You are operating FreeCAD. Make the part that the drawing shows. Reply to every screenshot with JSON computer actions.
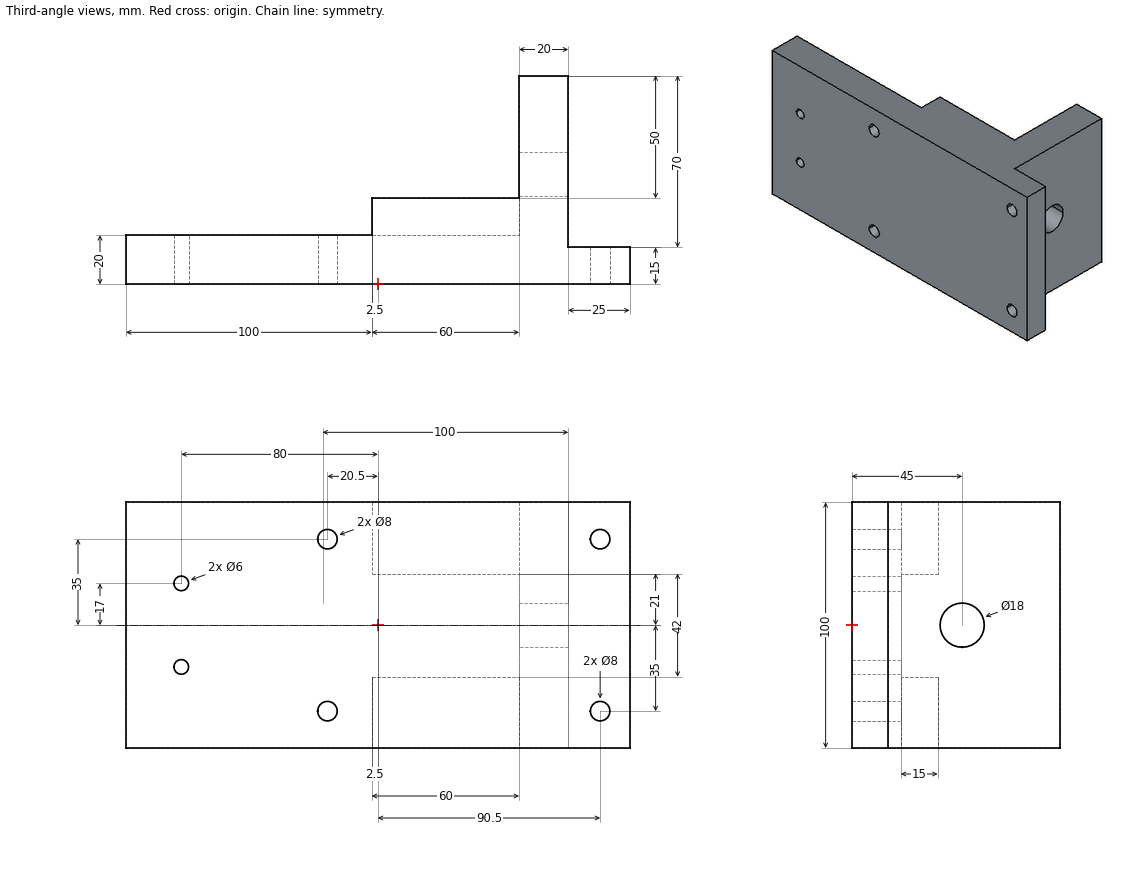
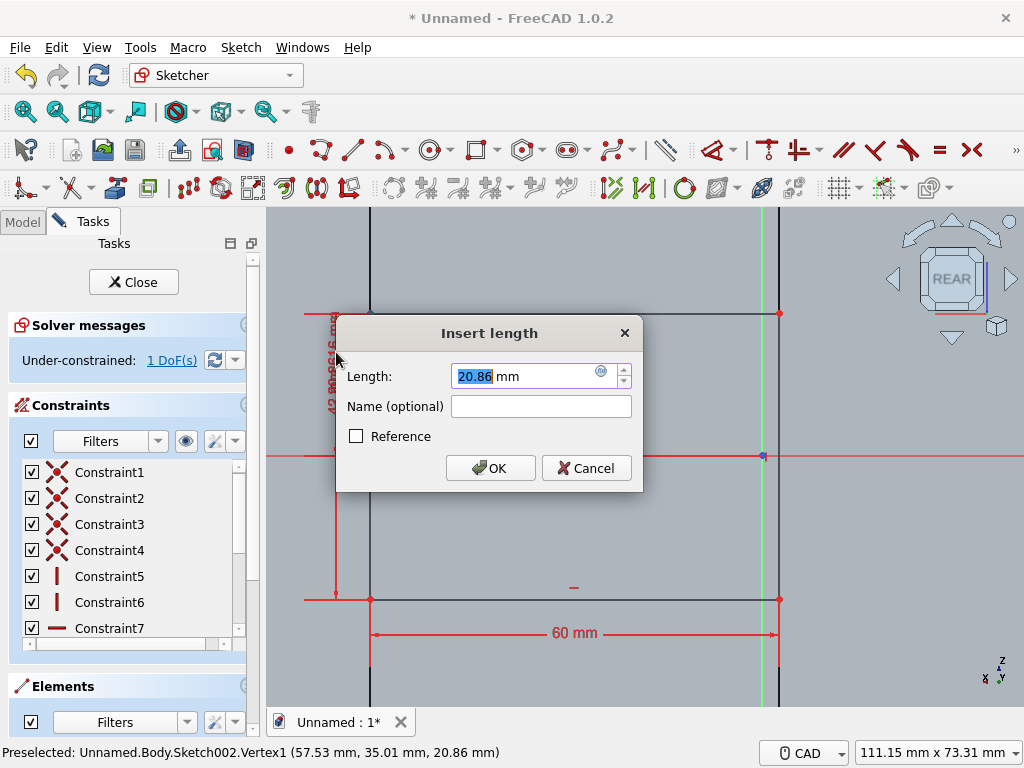
{"action": "type", "text": "21"}
{"action": "key", "text": "Return"}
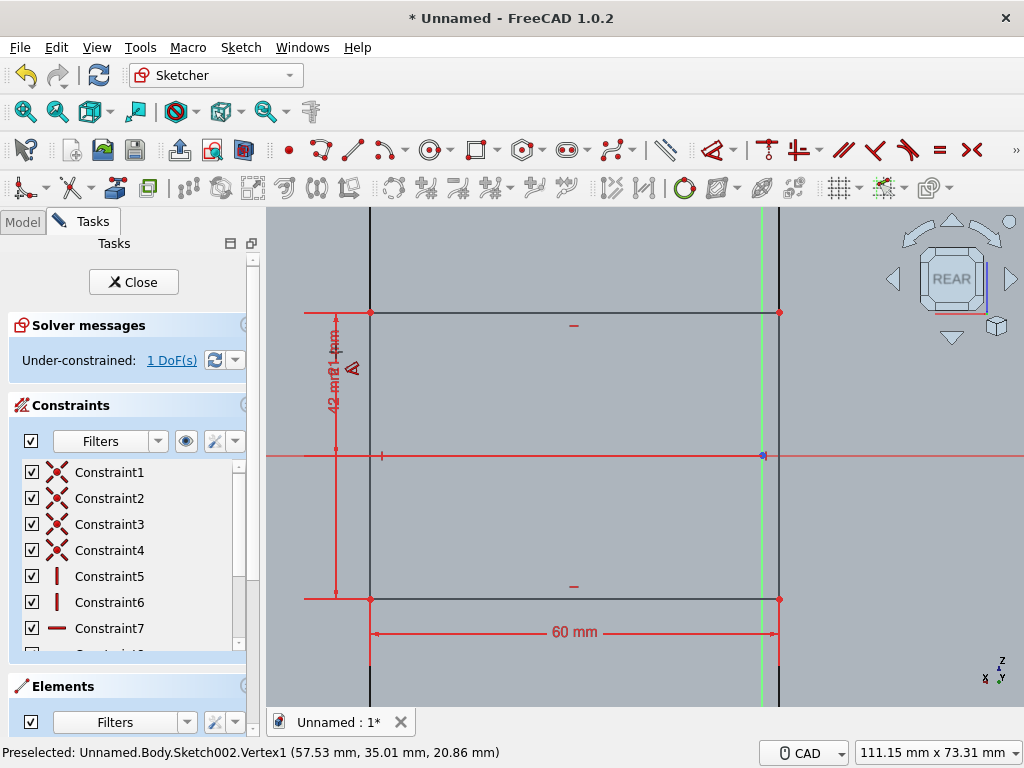
{"action": "scroll", "coordinate": [779, 599], "scroll_direction": "up", "scroll_amount": 5}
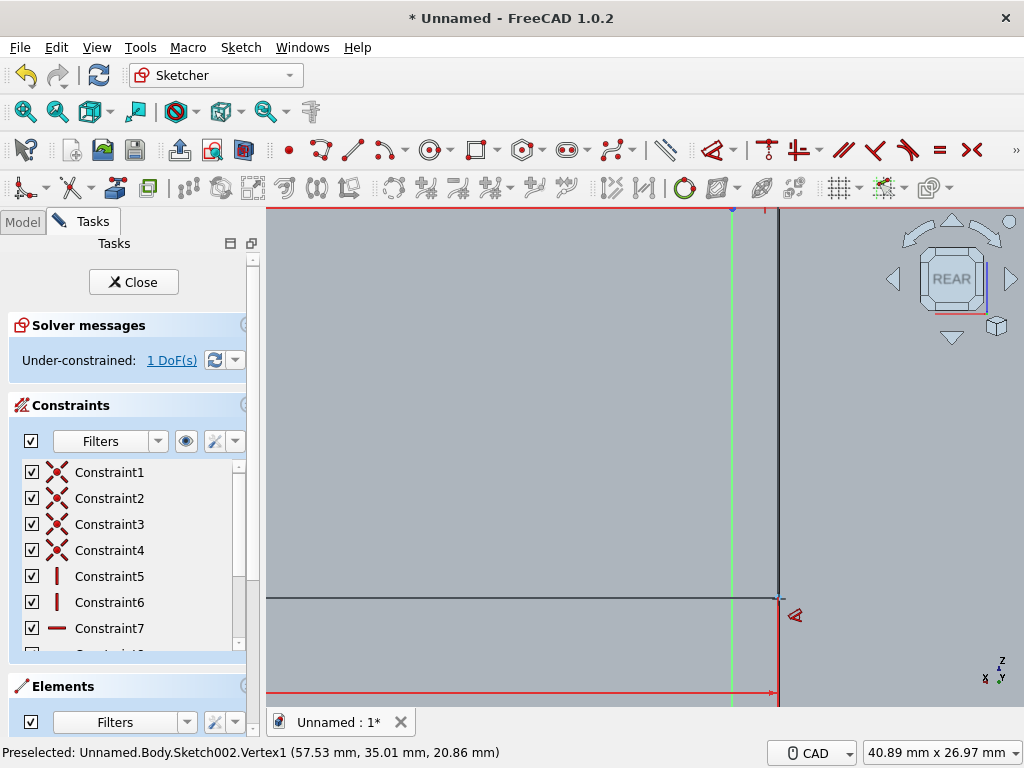
{"action": "left_click", "coordinate": [778, 598]}
{"action": "left_click", "coordinate": [755, 632]}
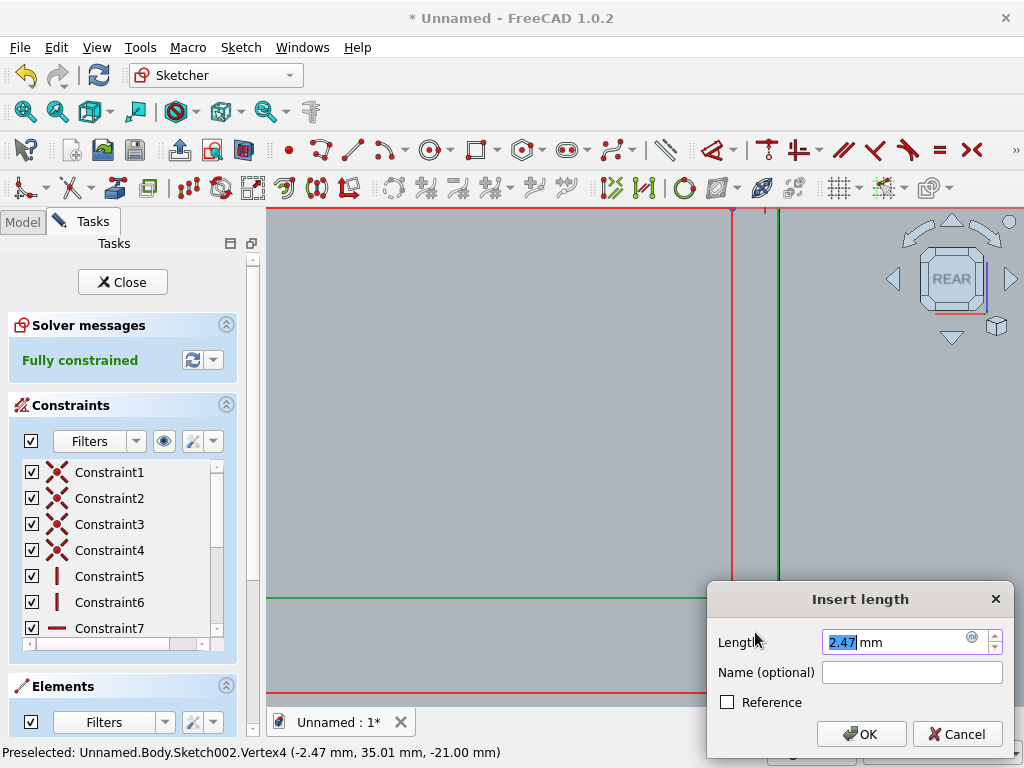
{"action": "type", "text": "2.5"}
{"action": "key", "text": "Return"}
{"action": "key", "text": "Escape"}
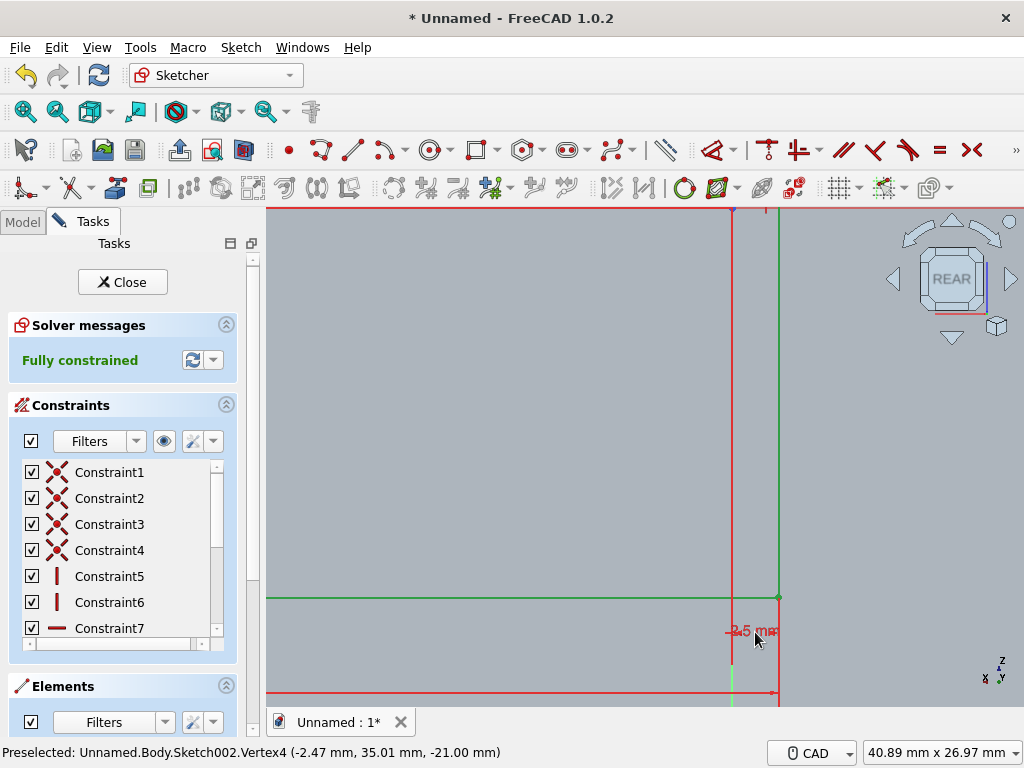
{"action": "left_click", "coordinate": [123, 282]}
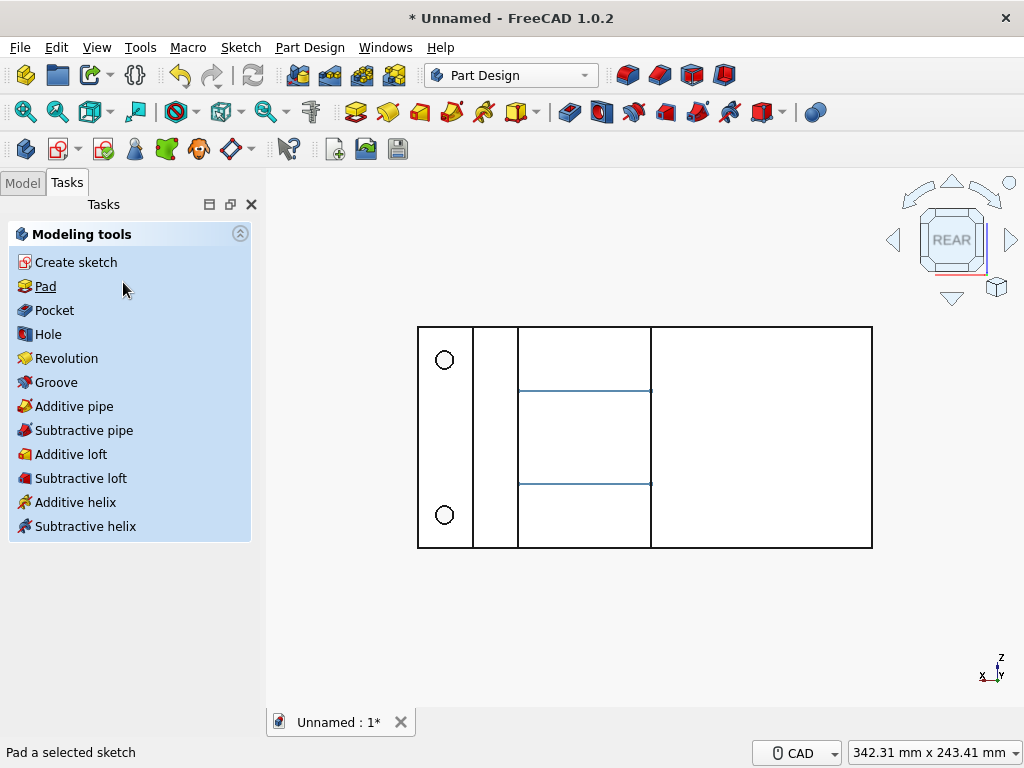
{"action": "left_click", "coordinate": [570, 112]}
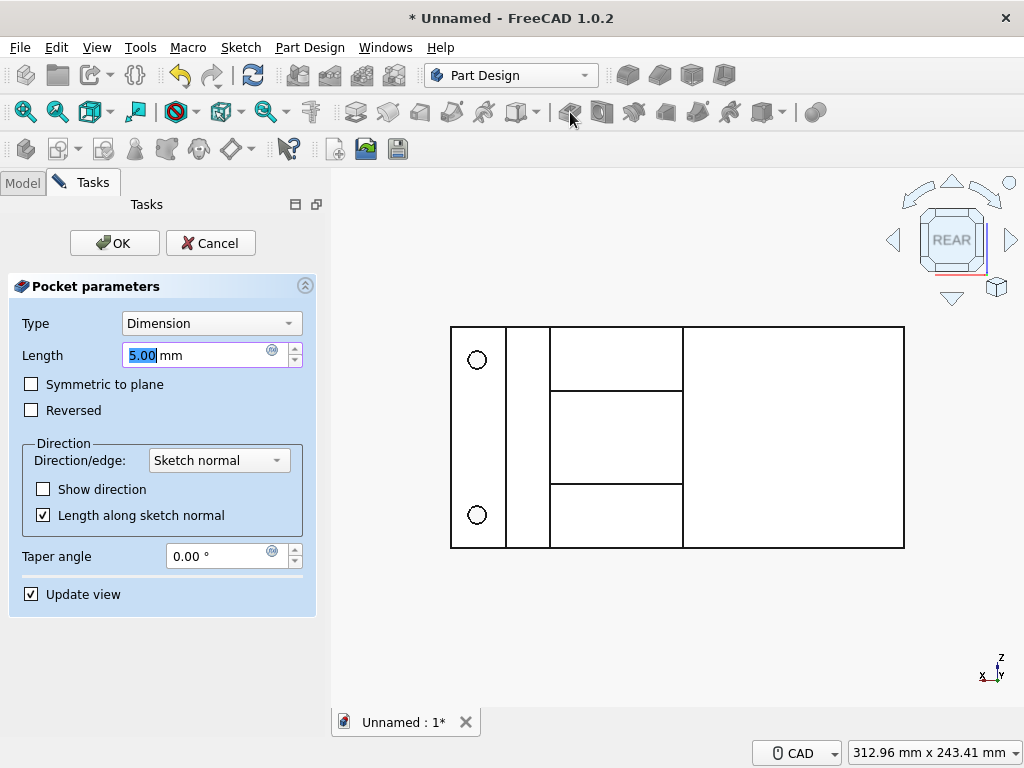
{"action": "type", "text": "15"}
{"action": "key", "text": "Tab"}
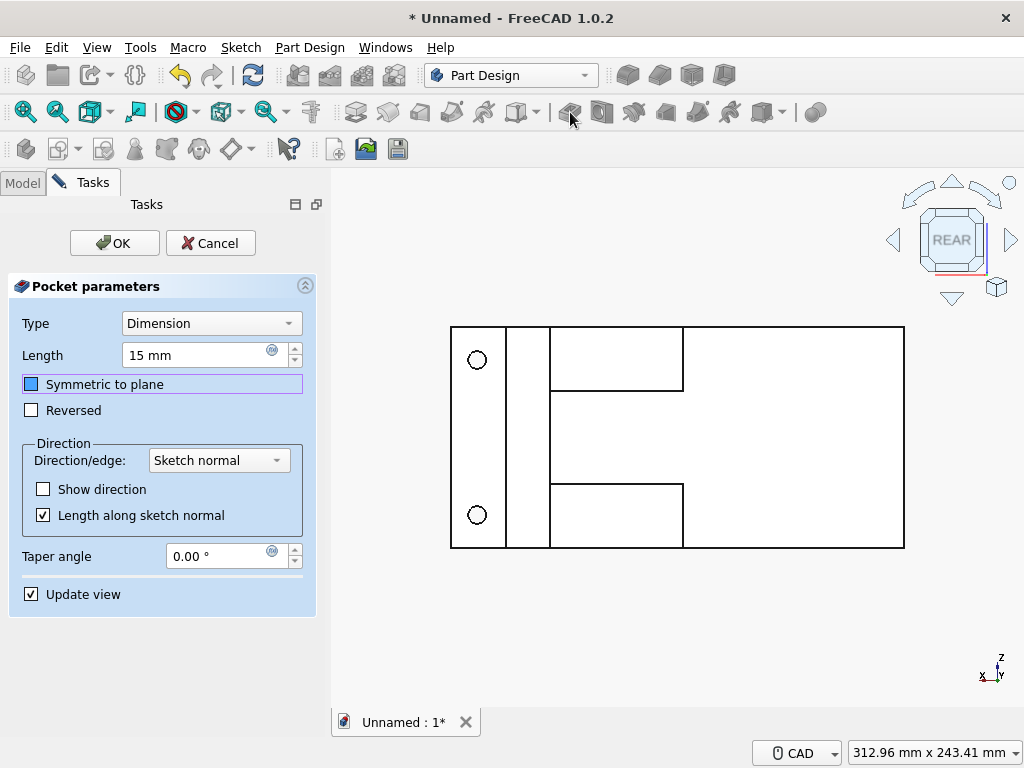
{"action": "left_click", "coordinate": [115, 243]}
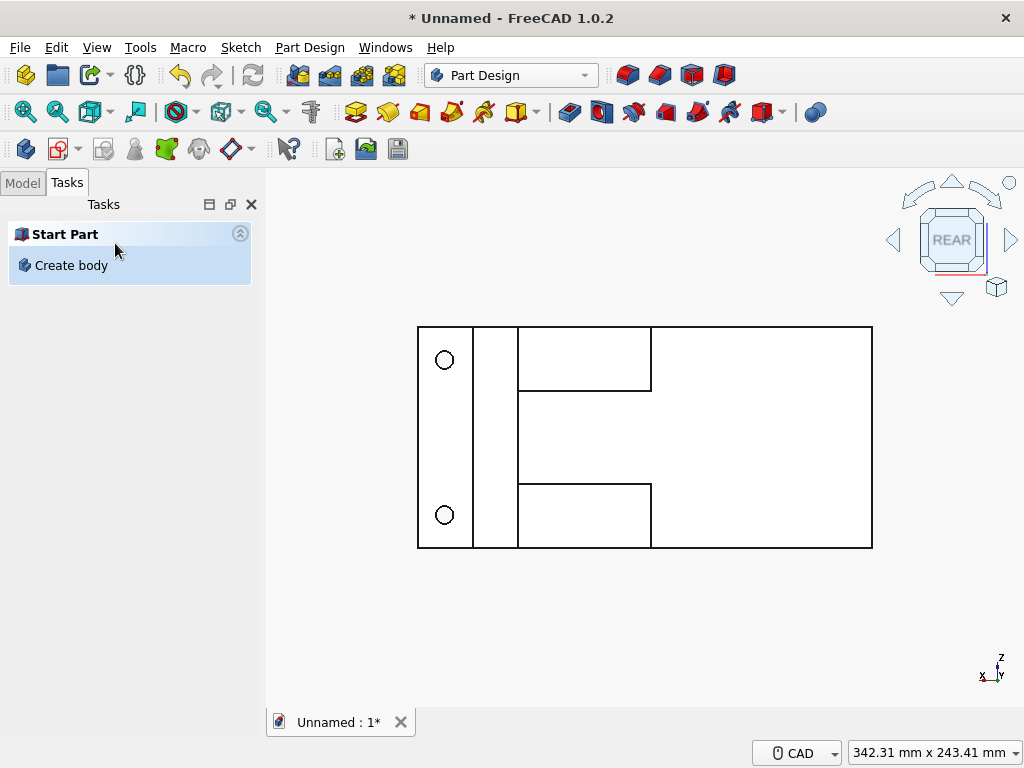
{"action": "key", "text": "0"}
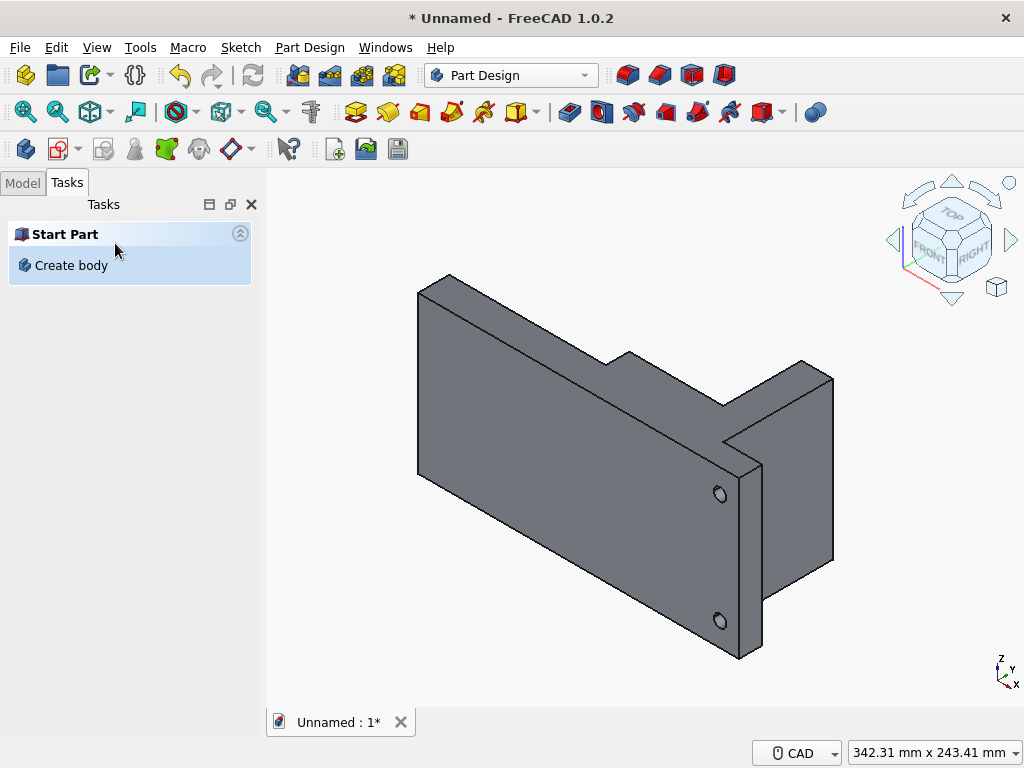
{"action": "left_click", "coordinate": [778, 474]}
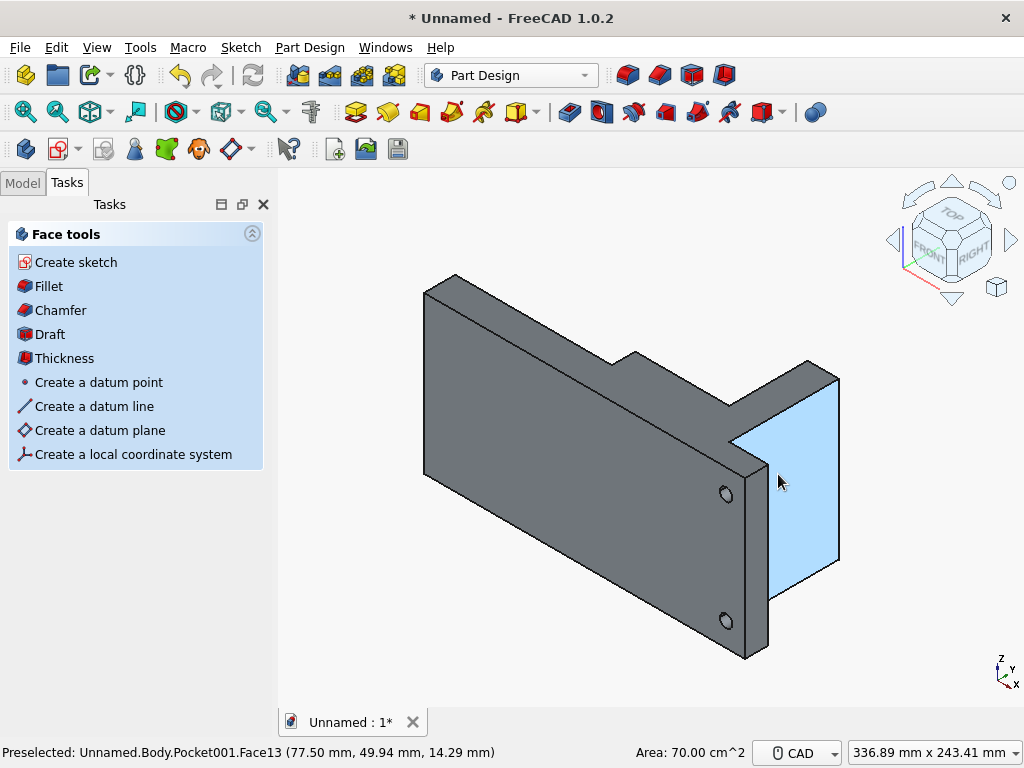
{"action": "left_click", "coordinate": [58, 150]}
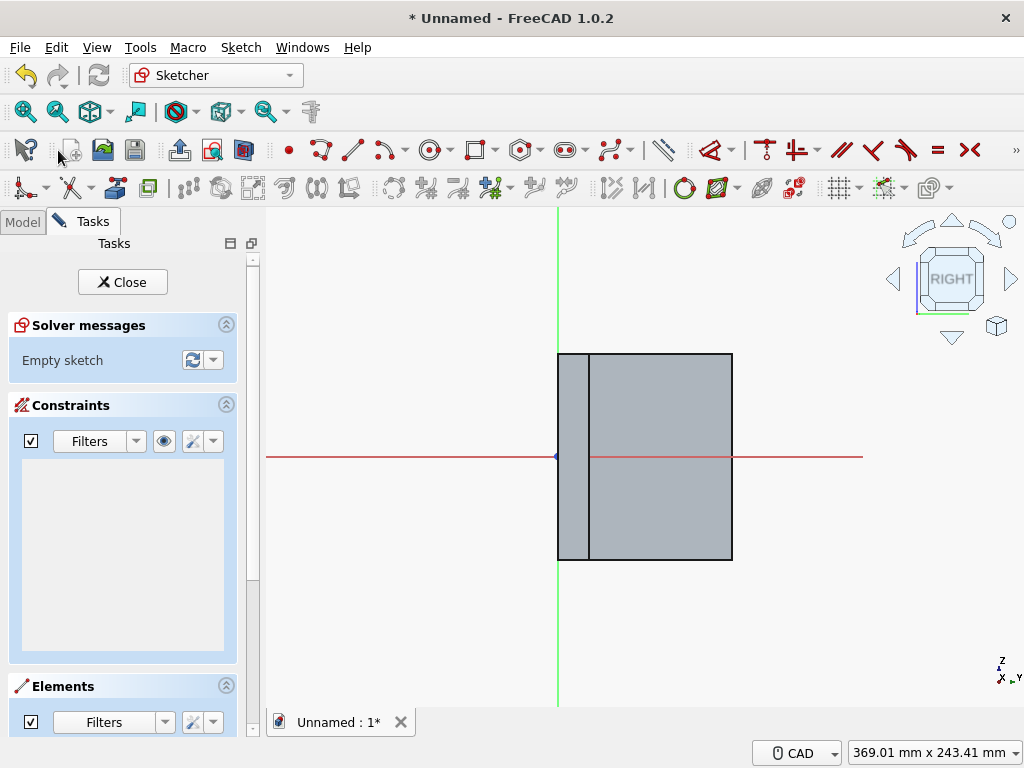
{"action": "scroll", "coordinate": [659, 457], "scroll_direction": "up", "scroll_amount": 11}